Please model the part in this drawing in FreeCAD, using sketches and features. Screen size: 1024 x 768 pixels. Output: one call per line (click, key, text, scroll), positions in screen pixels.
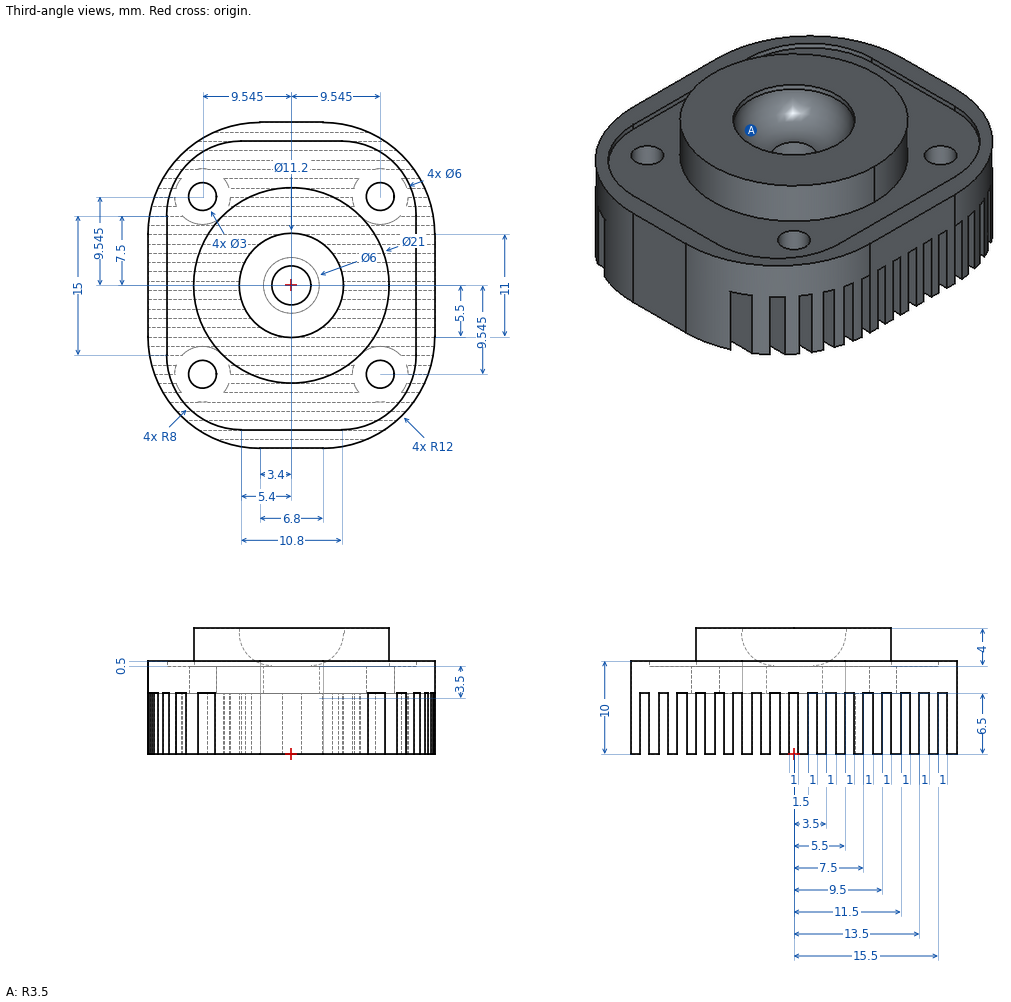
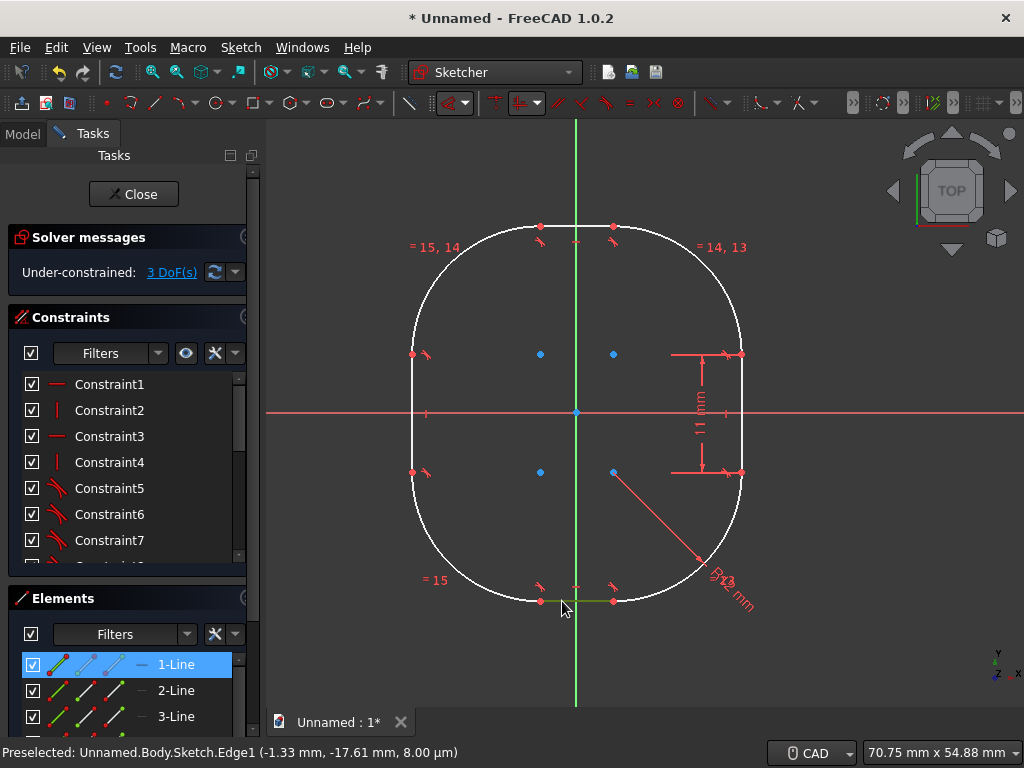
click(468, 104)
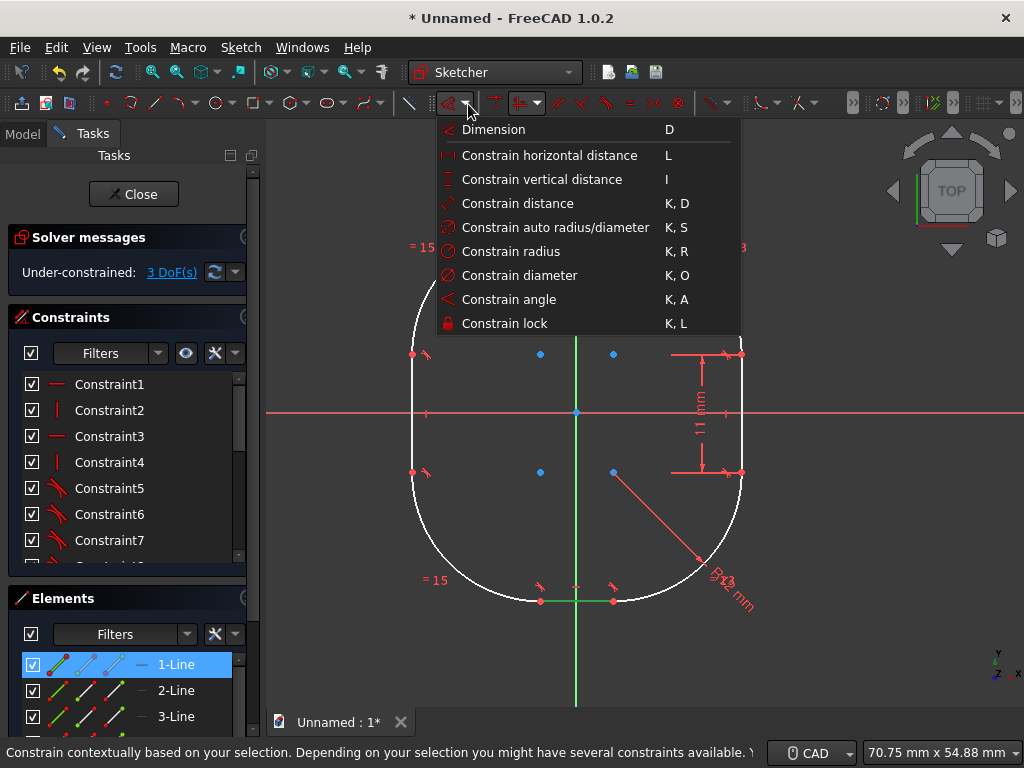
click(589, 155)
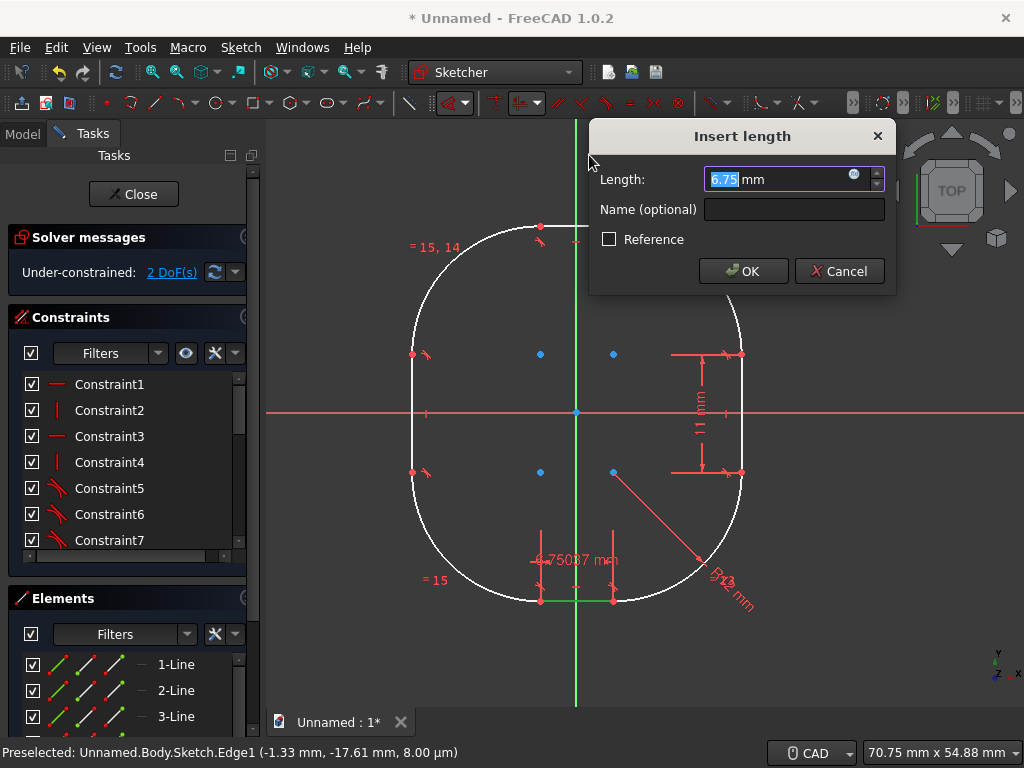
text(6.8)
key(Return)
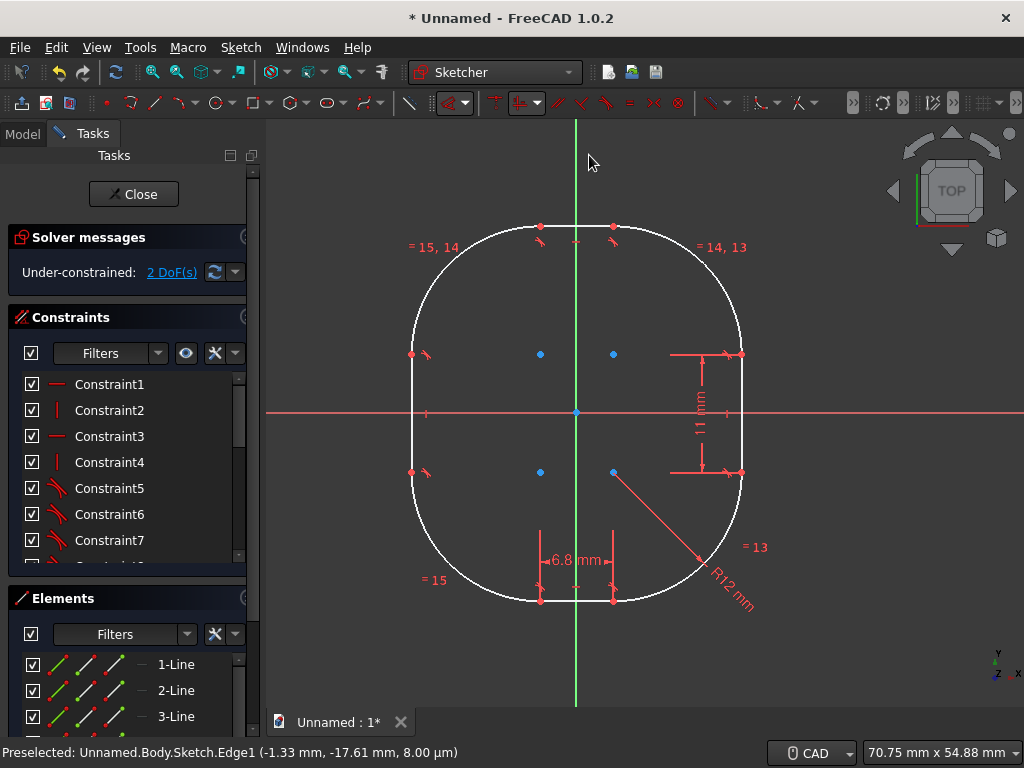
click(540, 601)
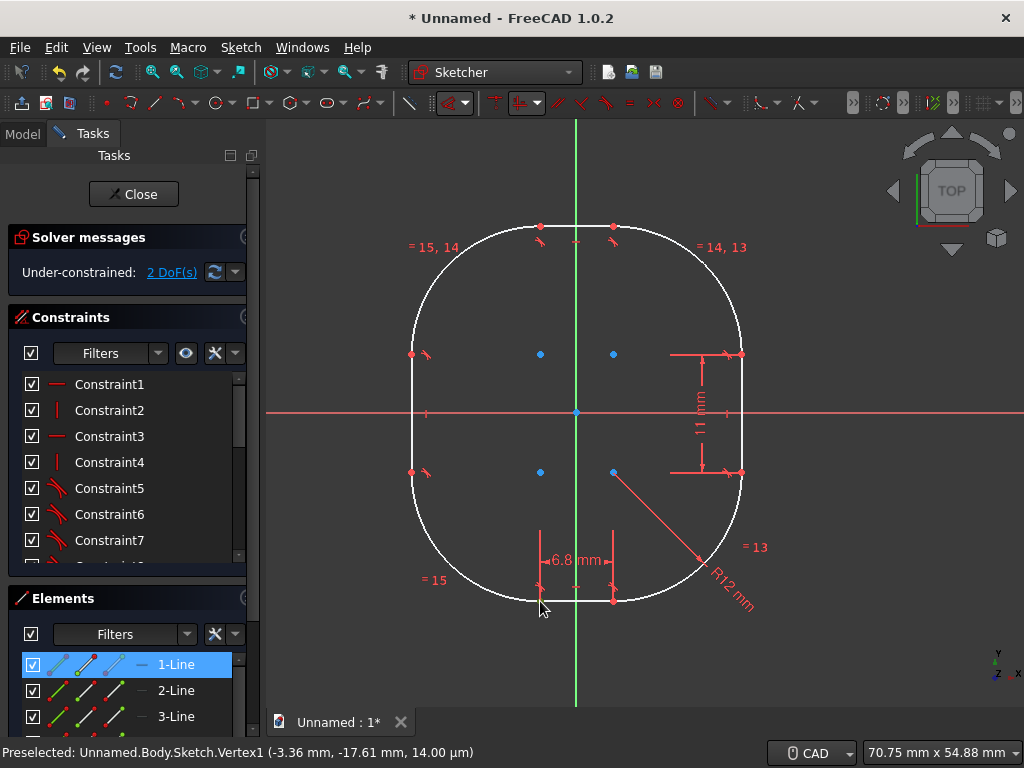
click(468, 104)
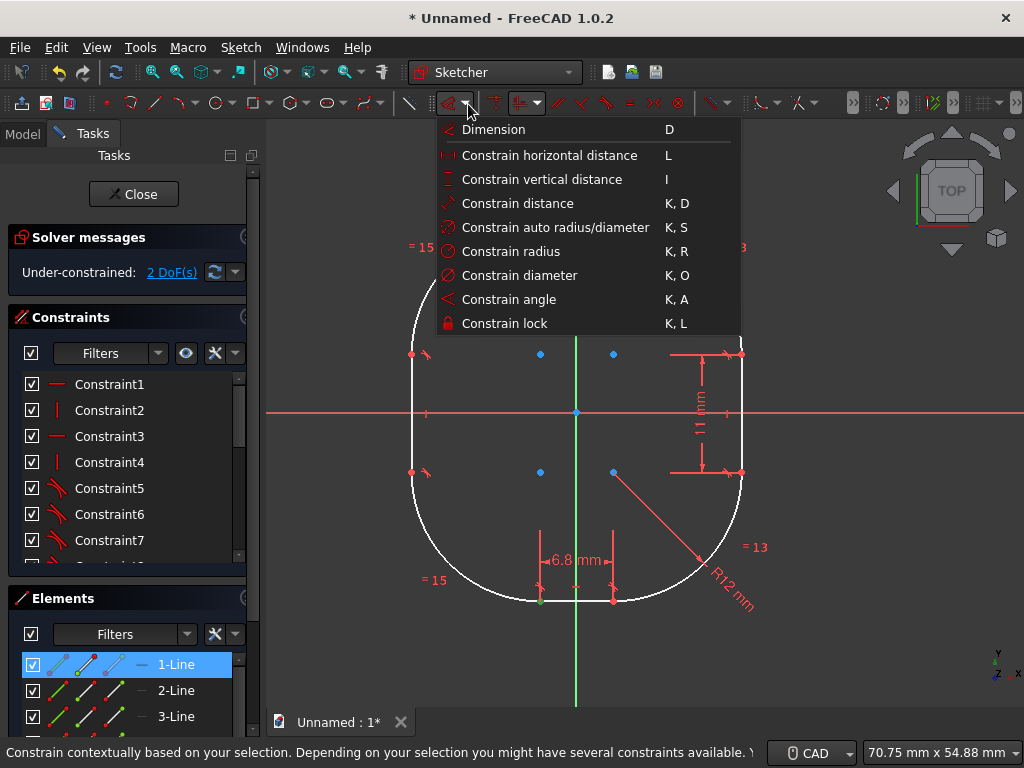
click(589, 155)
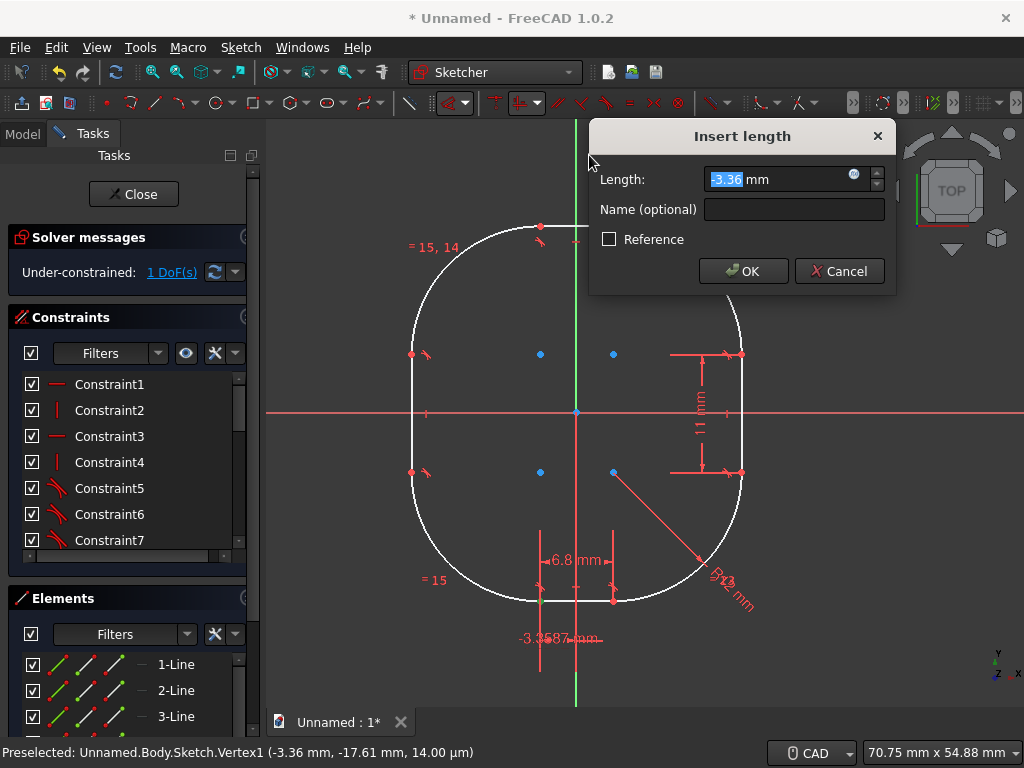
text(-3.4)
key(Return)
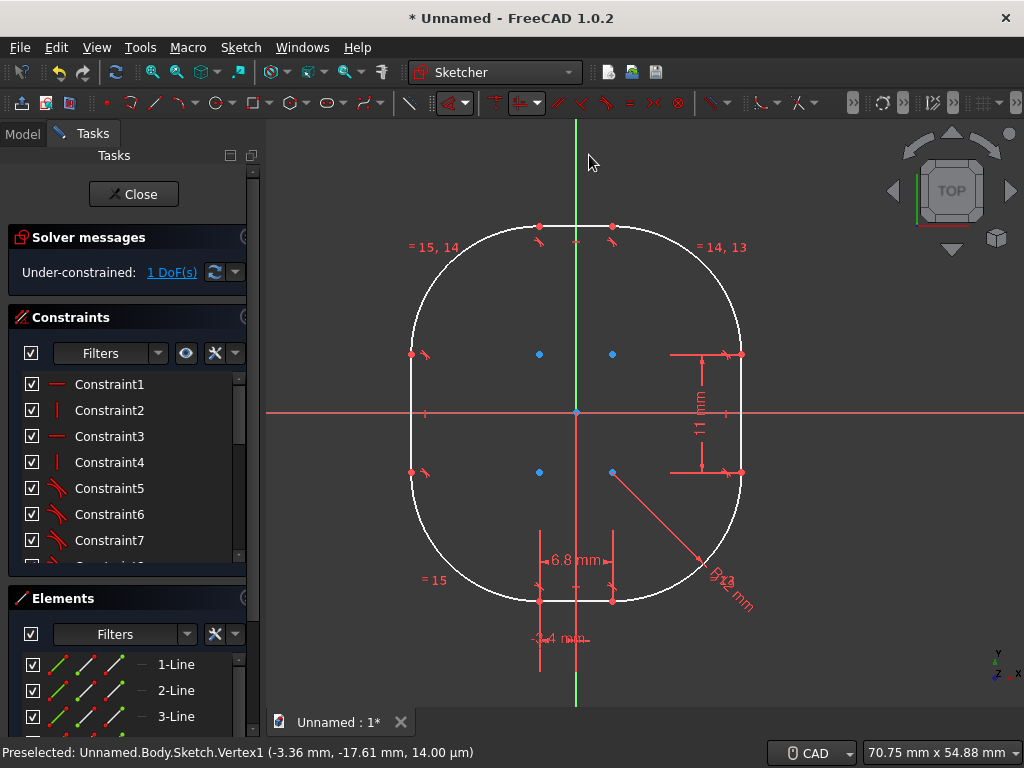
click(741, 473)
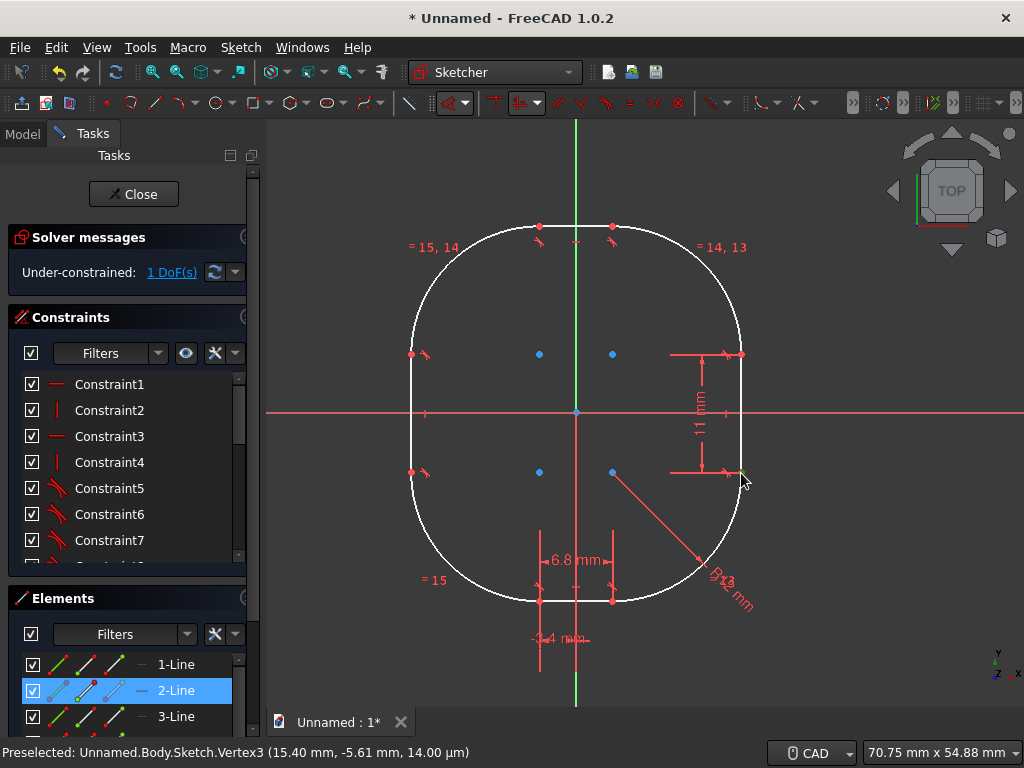
click(468, 104)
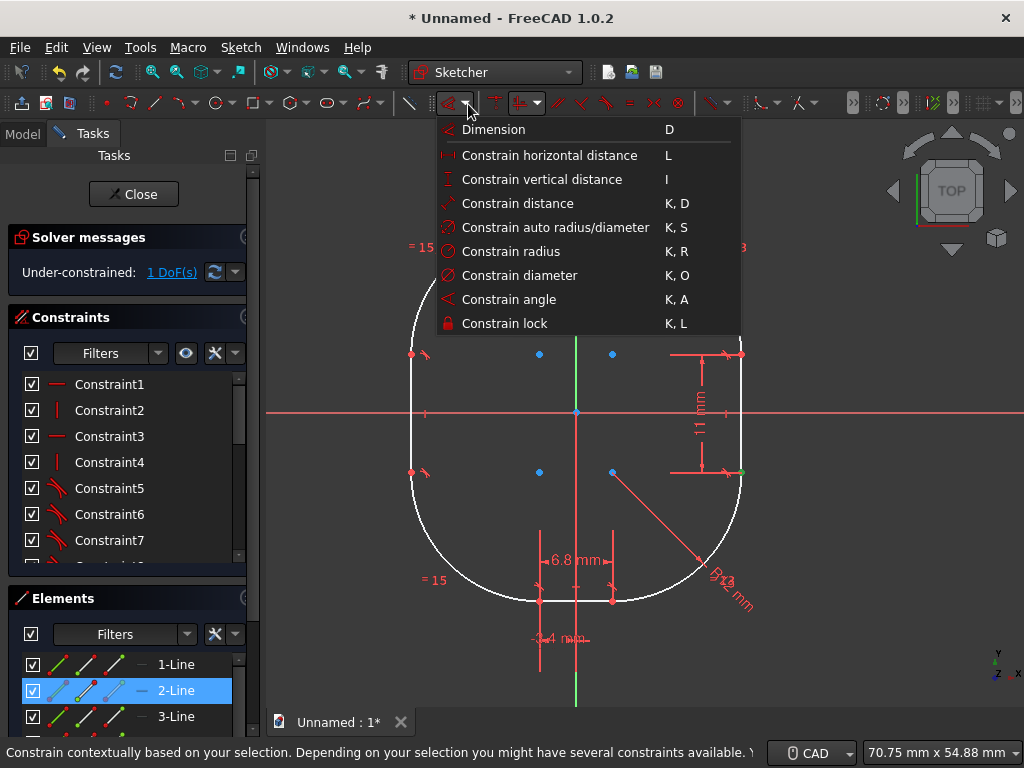
click(589, 179)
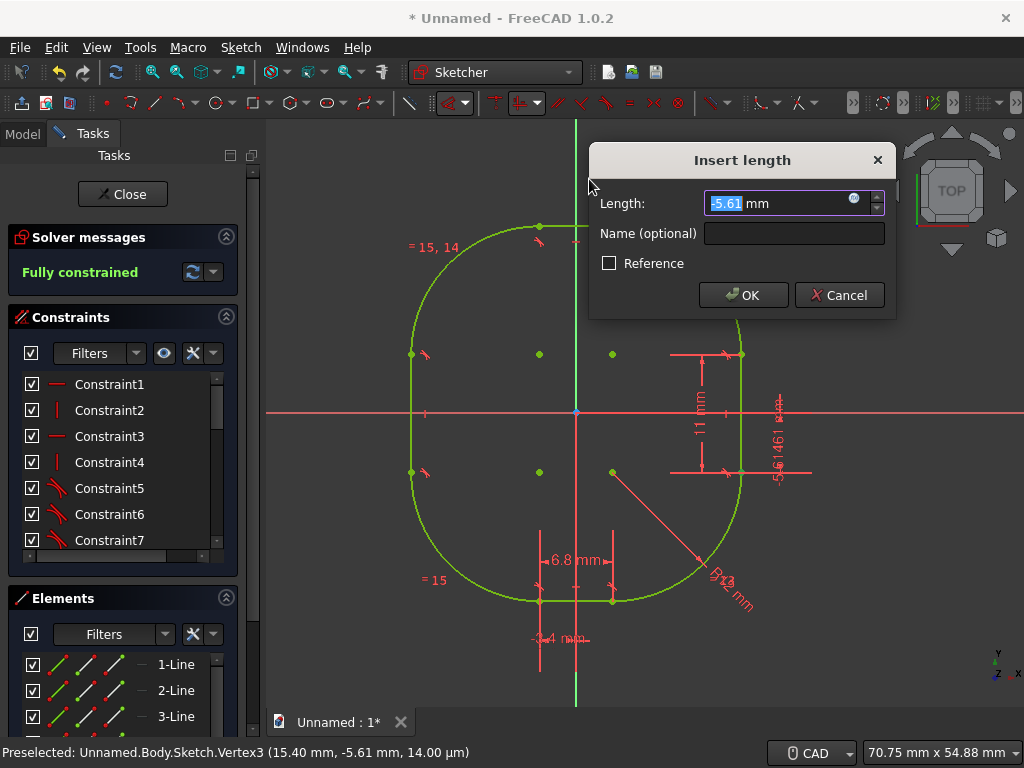
text(-5.5)
key(Return)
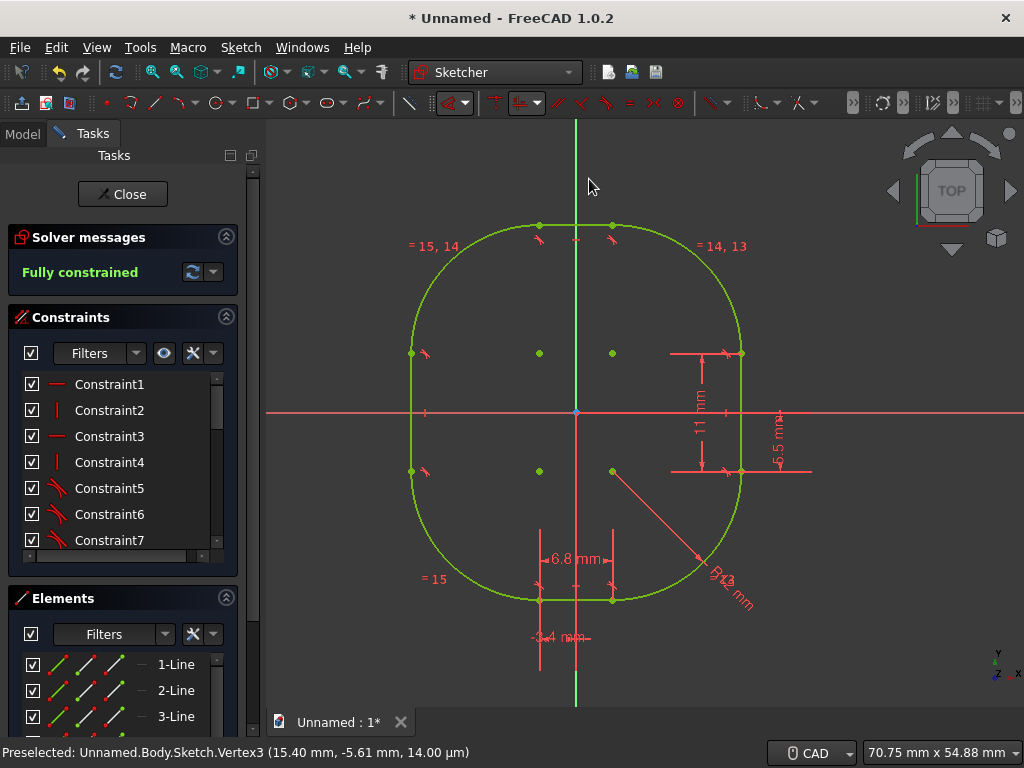
click(123, 194)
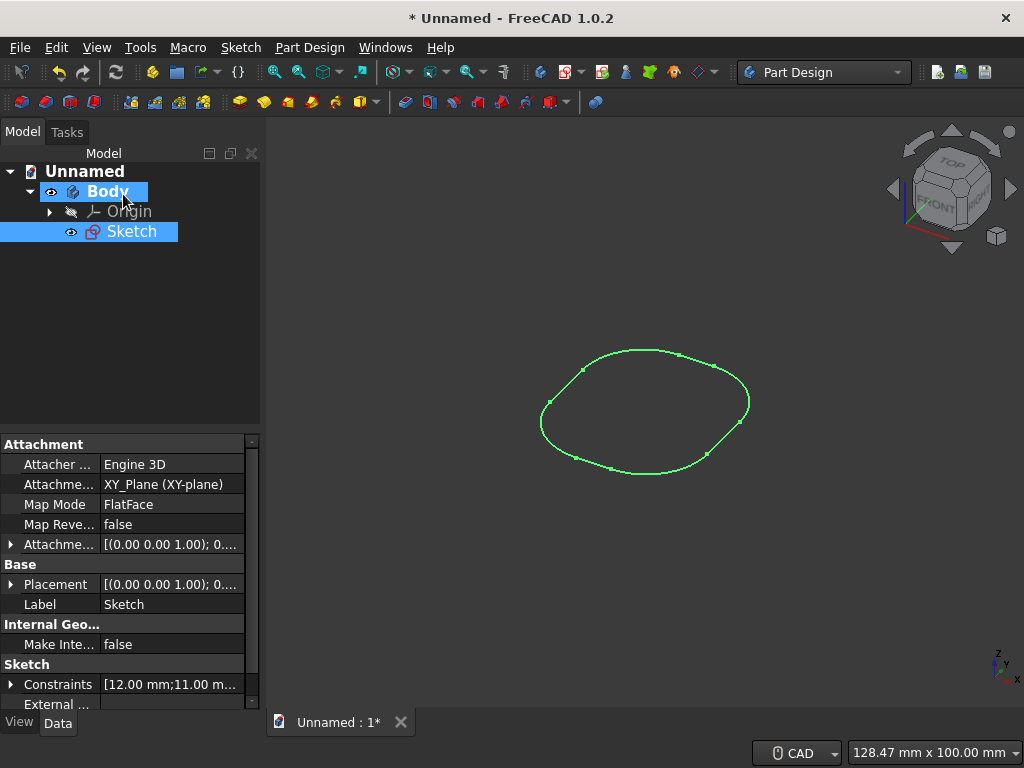
click(240, 102)